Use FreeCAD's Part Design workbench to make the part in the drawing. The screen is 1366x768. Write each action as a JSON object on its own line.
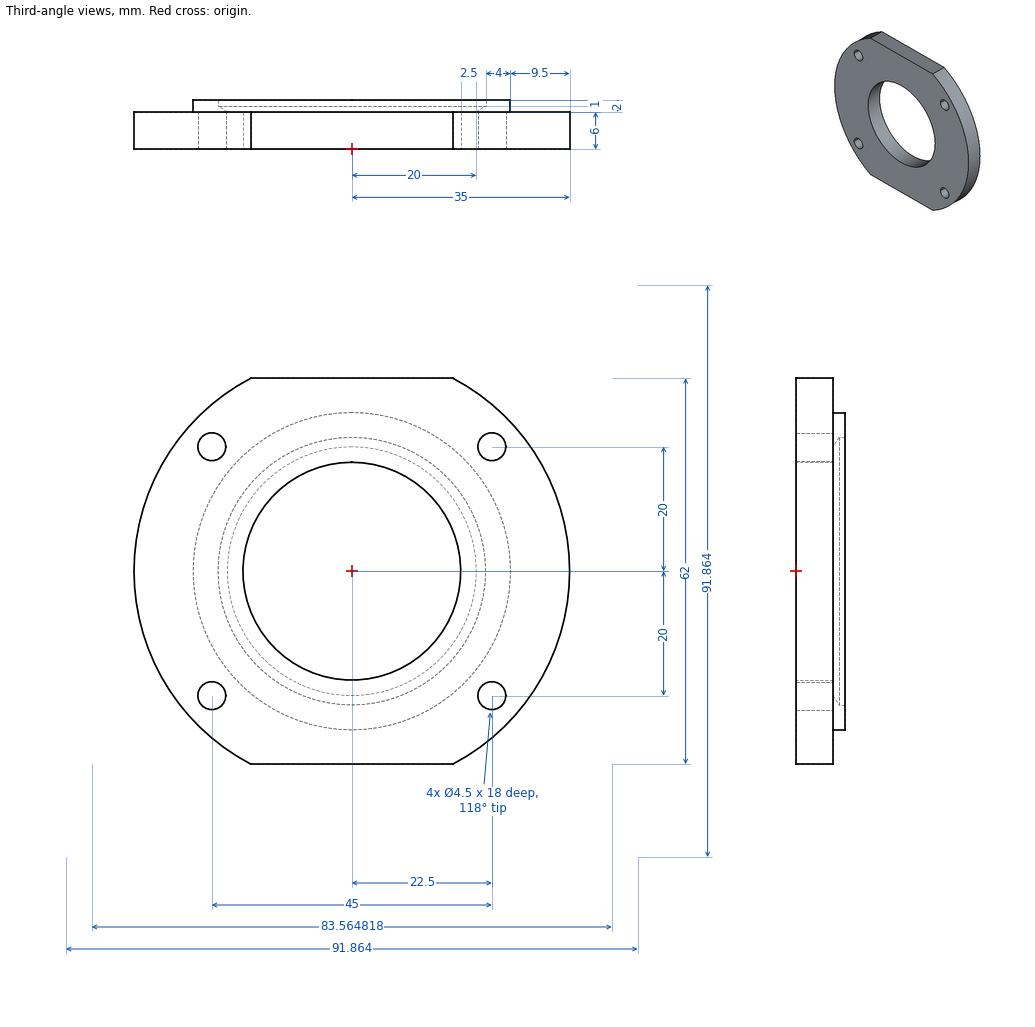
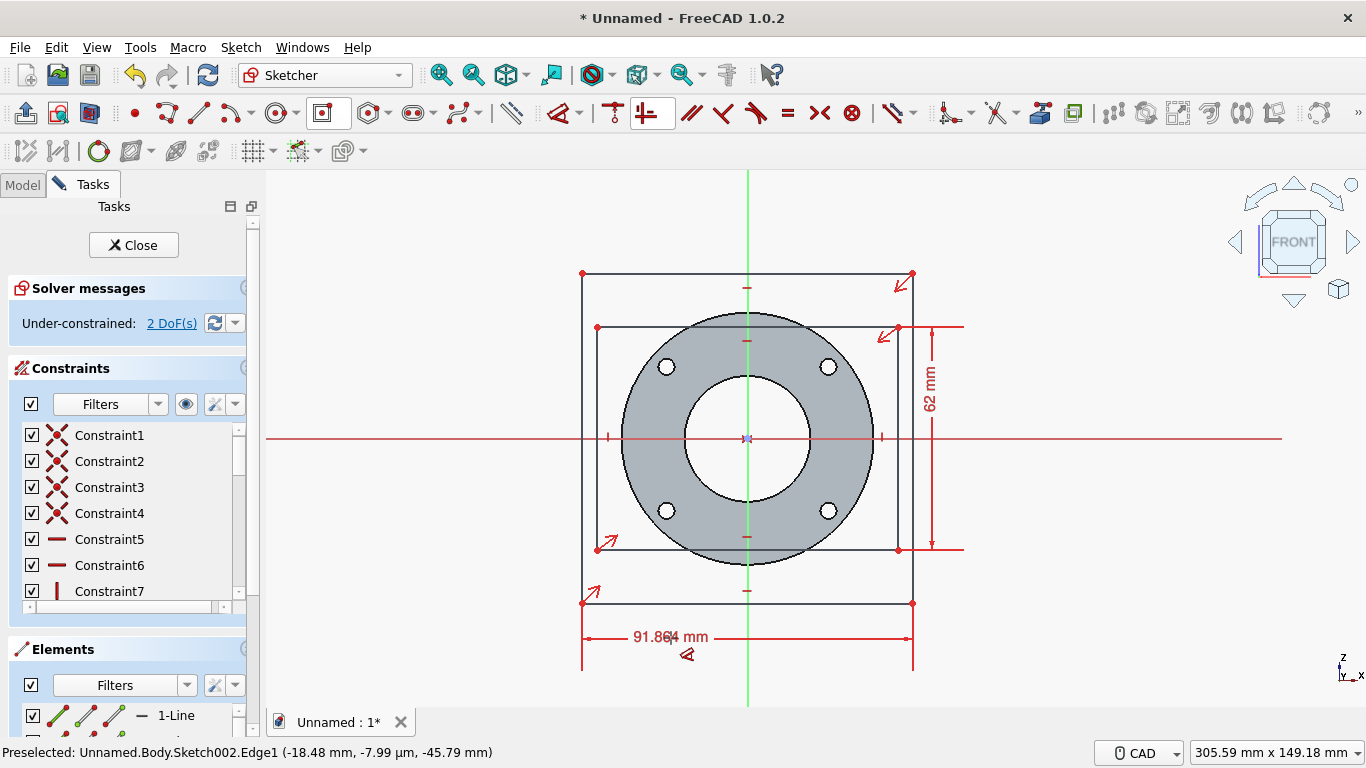
{"action": "left_click", "coordinate": [913, 505]}
{"action": "left_click", "coordinate": [947, 363]}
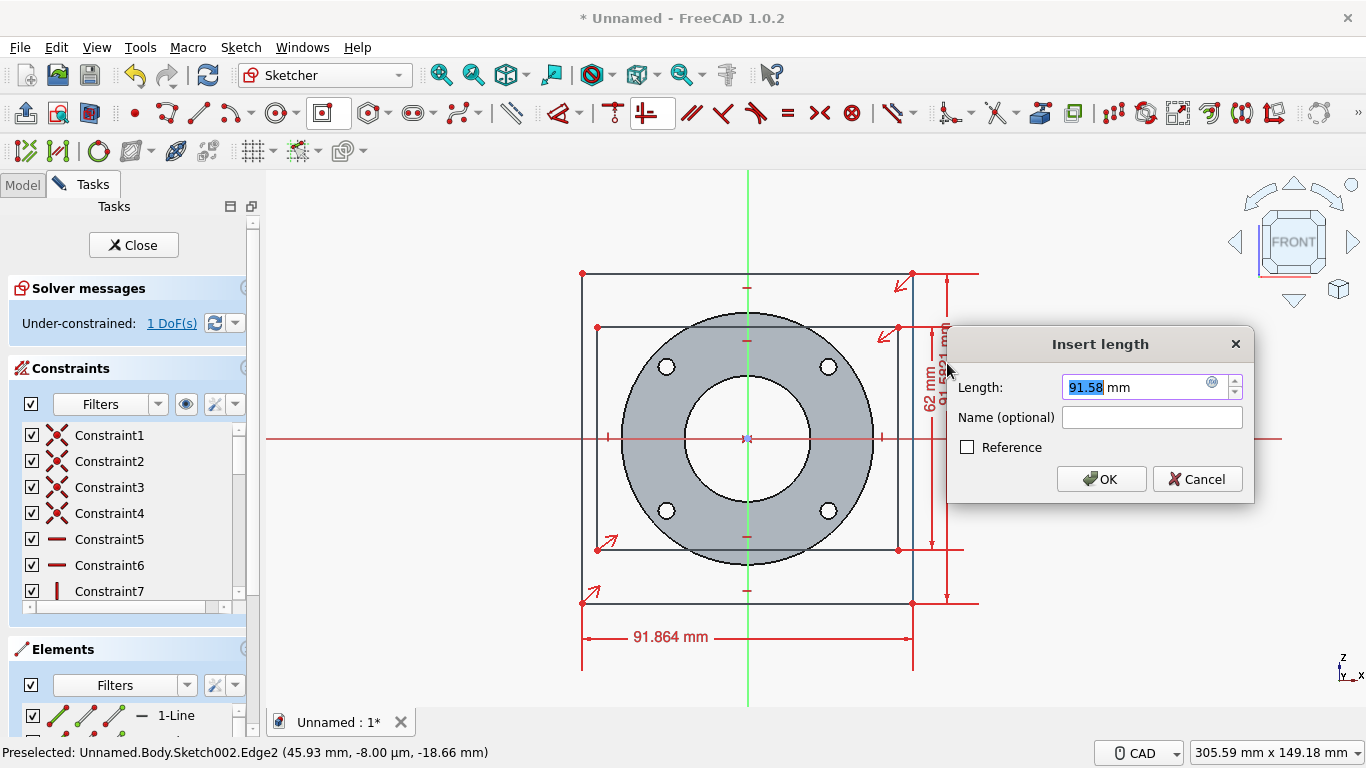
{"action": "type", "text": "91.864"}
{"action": "key", "text": "Return"}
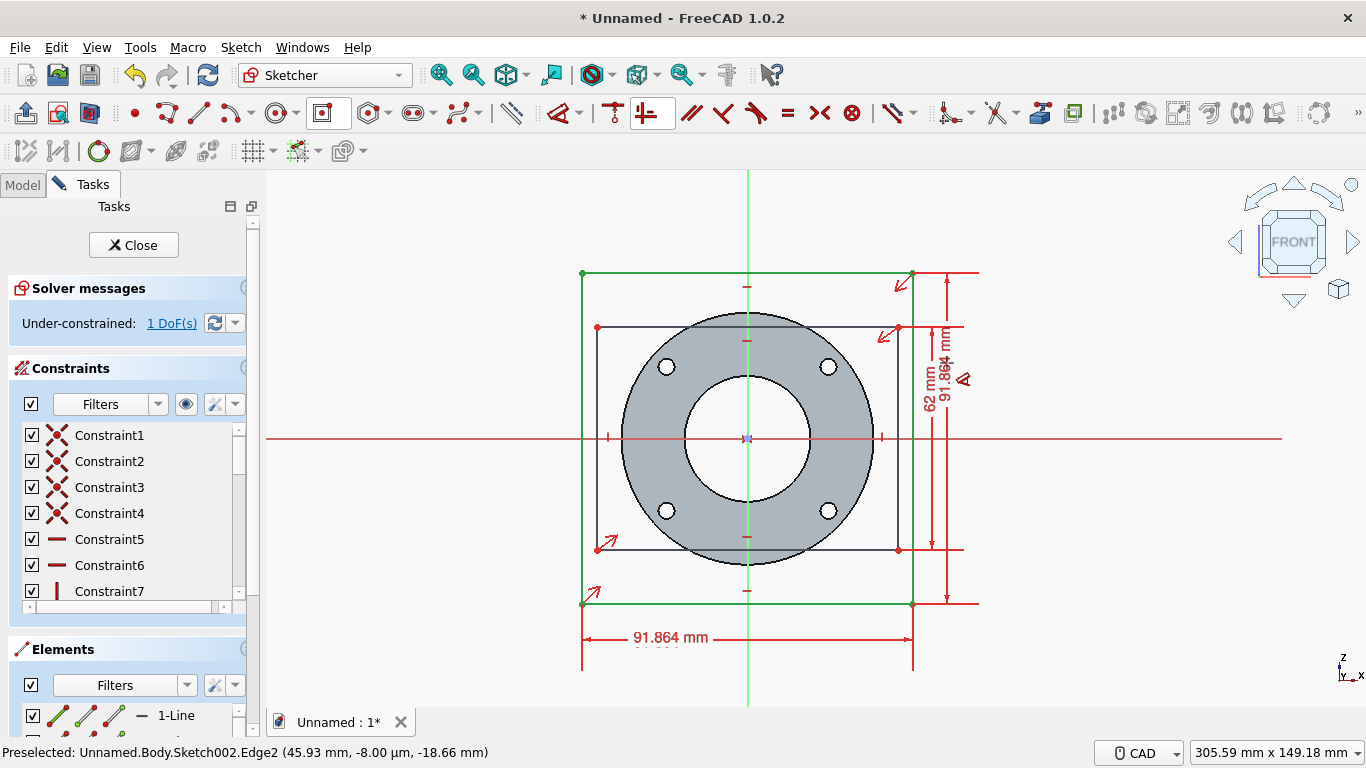
{"action": "left_click", "coordinate": [687, 550]}
{"action": "left_click", "coordinate": [678, 584]}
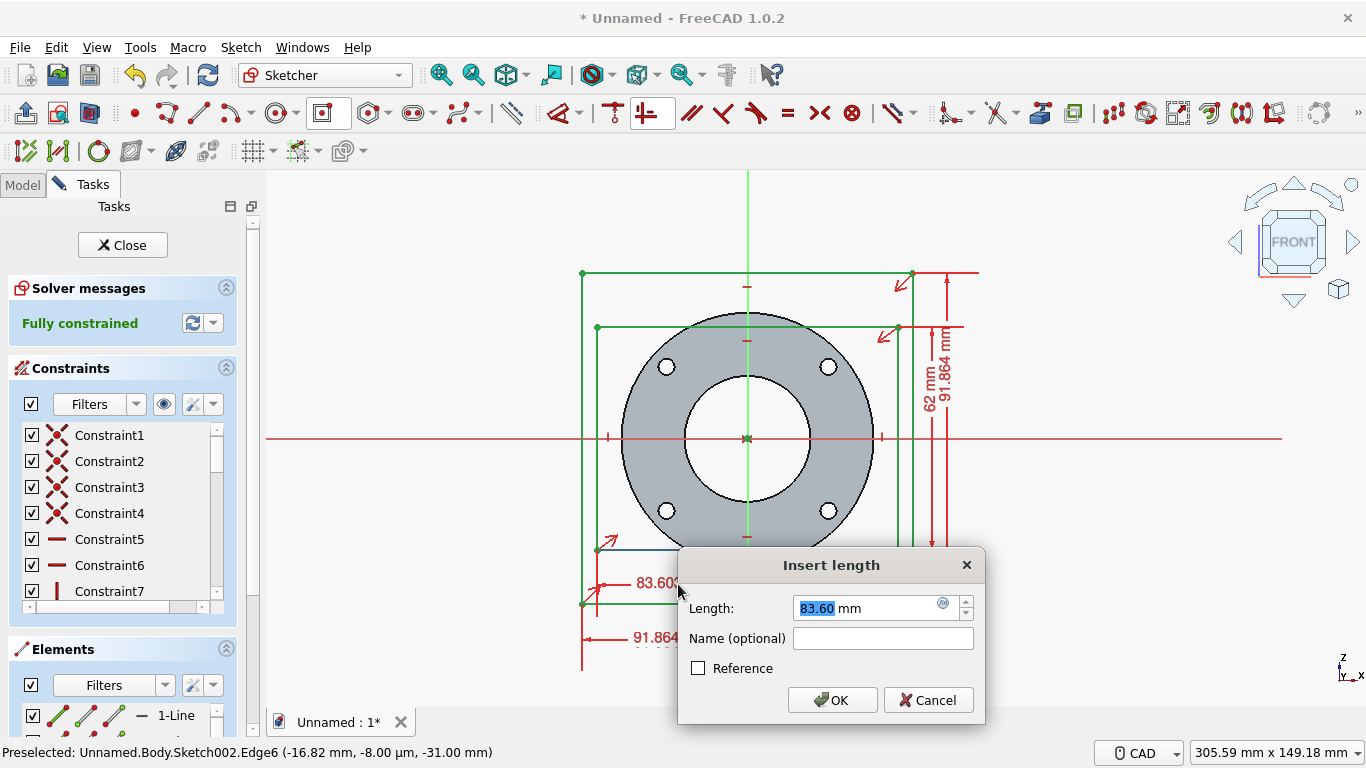
{"action": "type", "text": "83.564818"}
{"action": "key", "text": "Return"}
{"action": "key", "text": "Escape"}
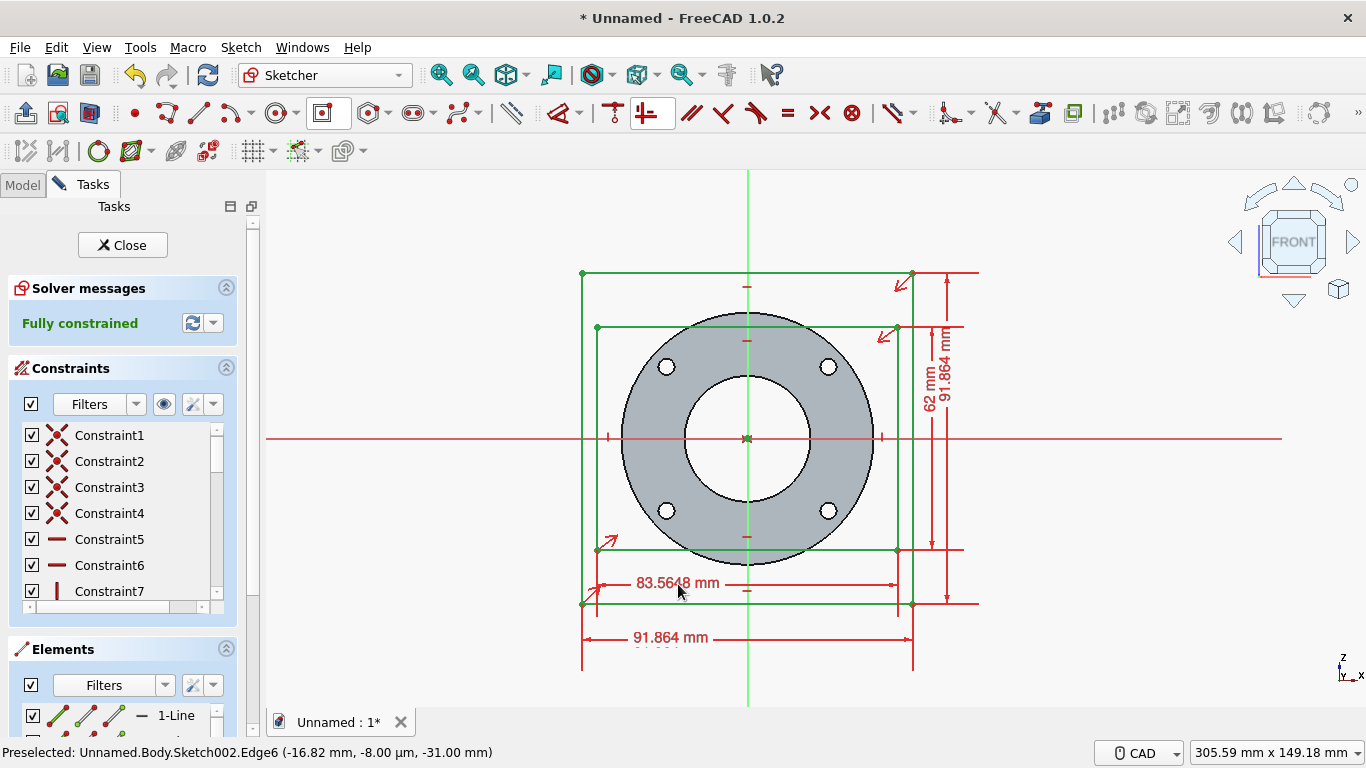
{"action": "left_click", "coordinate": [123, 245]}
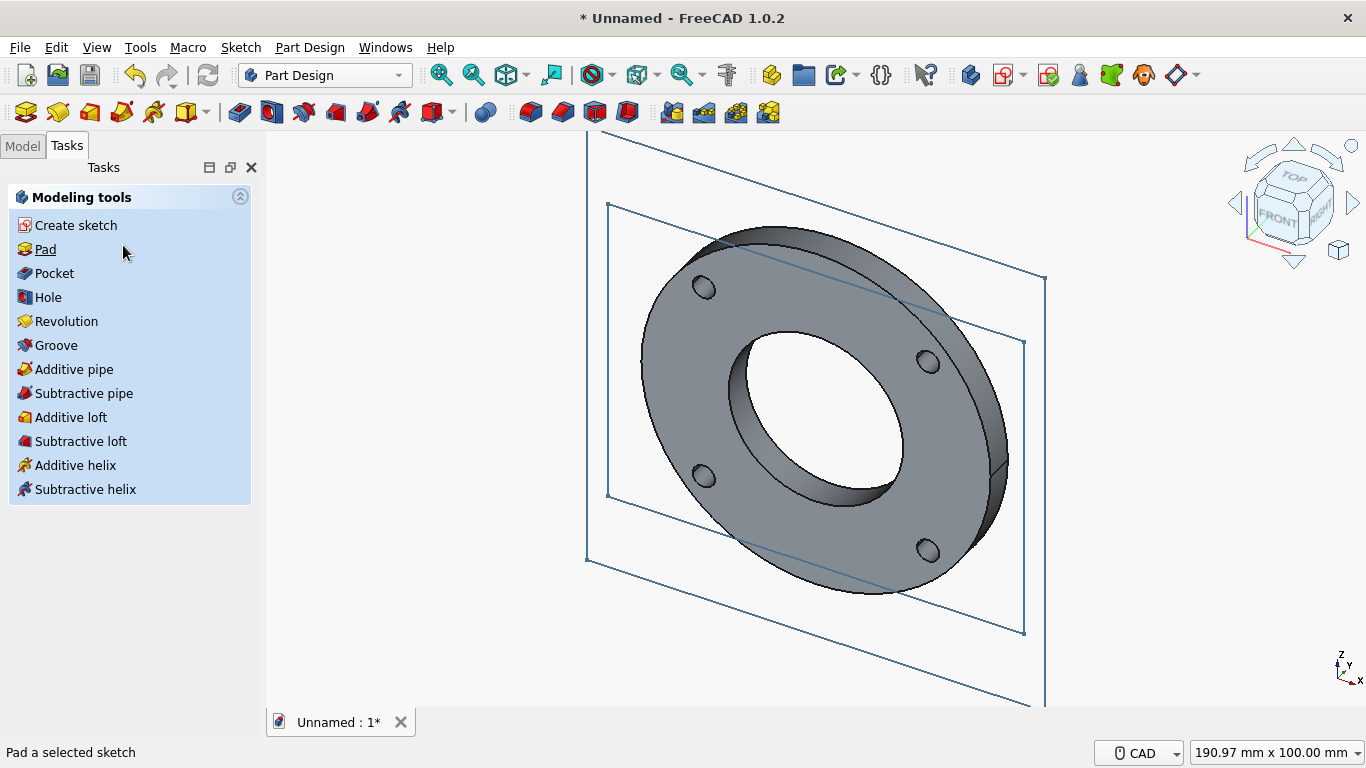
{"action": "left_click", "coordinate": [240, 112]}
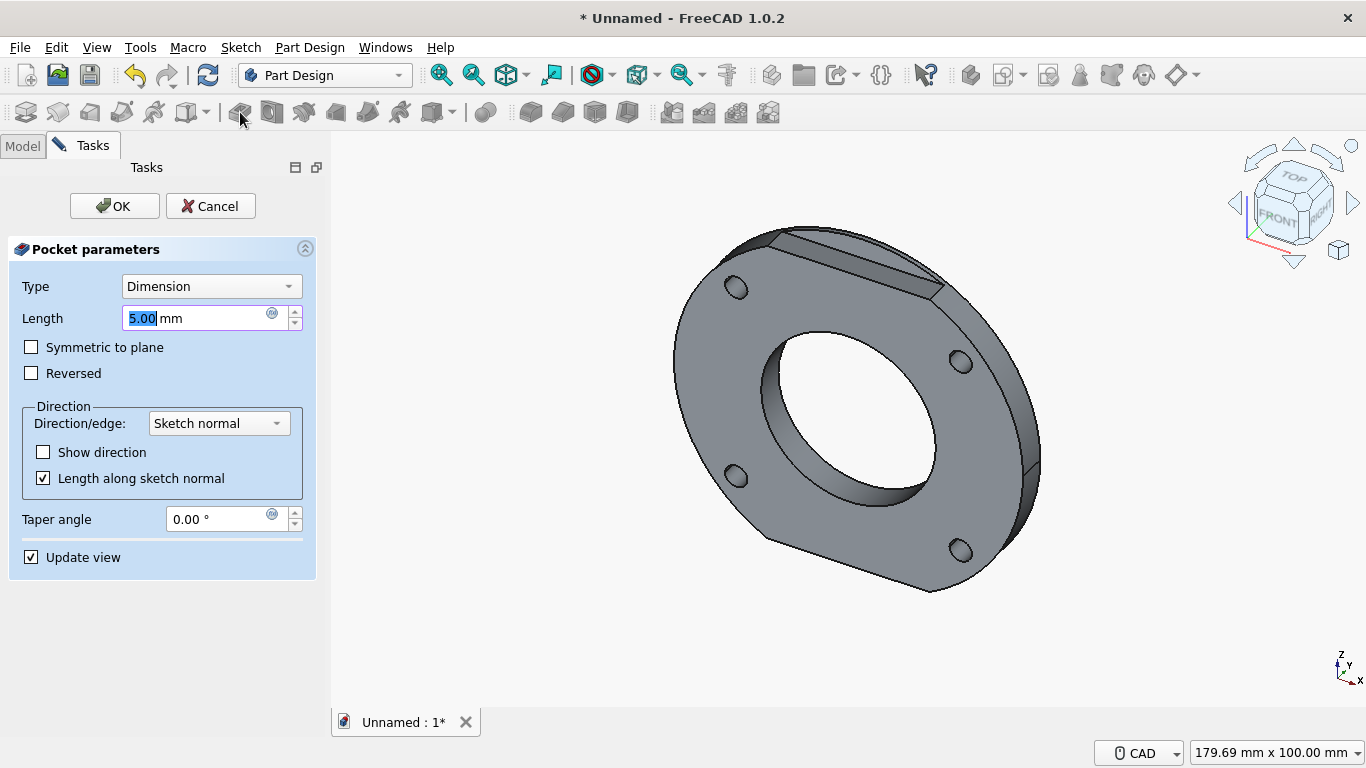
{"action": "left_click", "coordinate": [212, 286]}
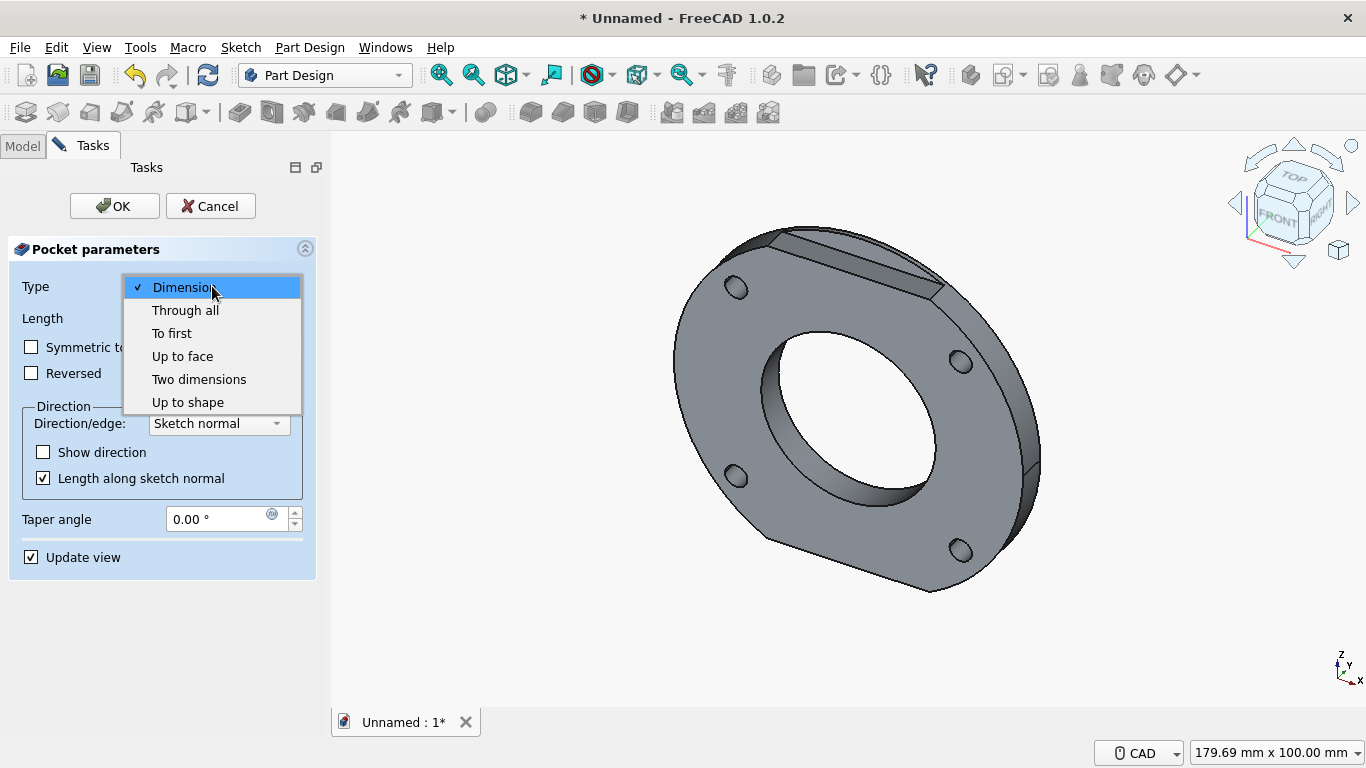
{"action": "left_click", "coordinate": [212, 310]}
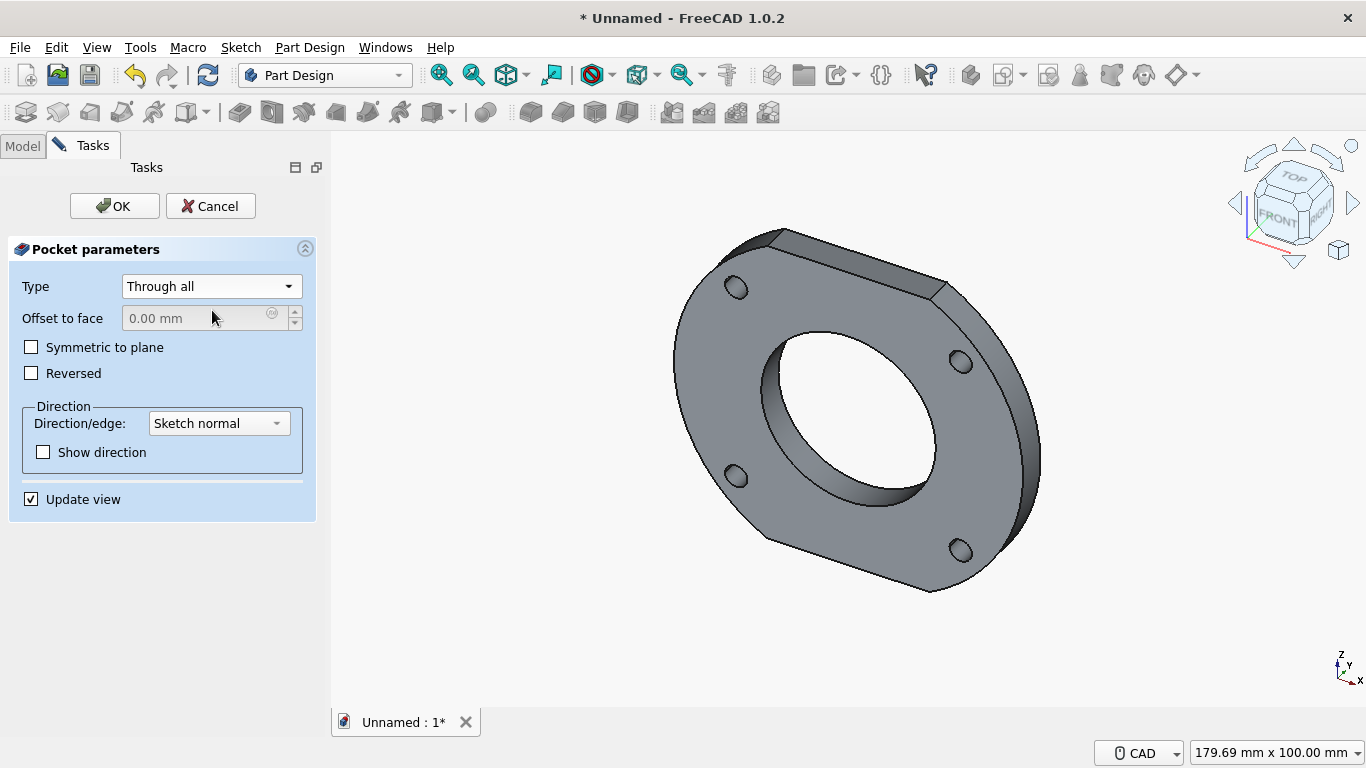
{"action": "left_click", "coordinate": [115, 206]}